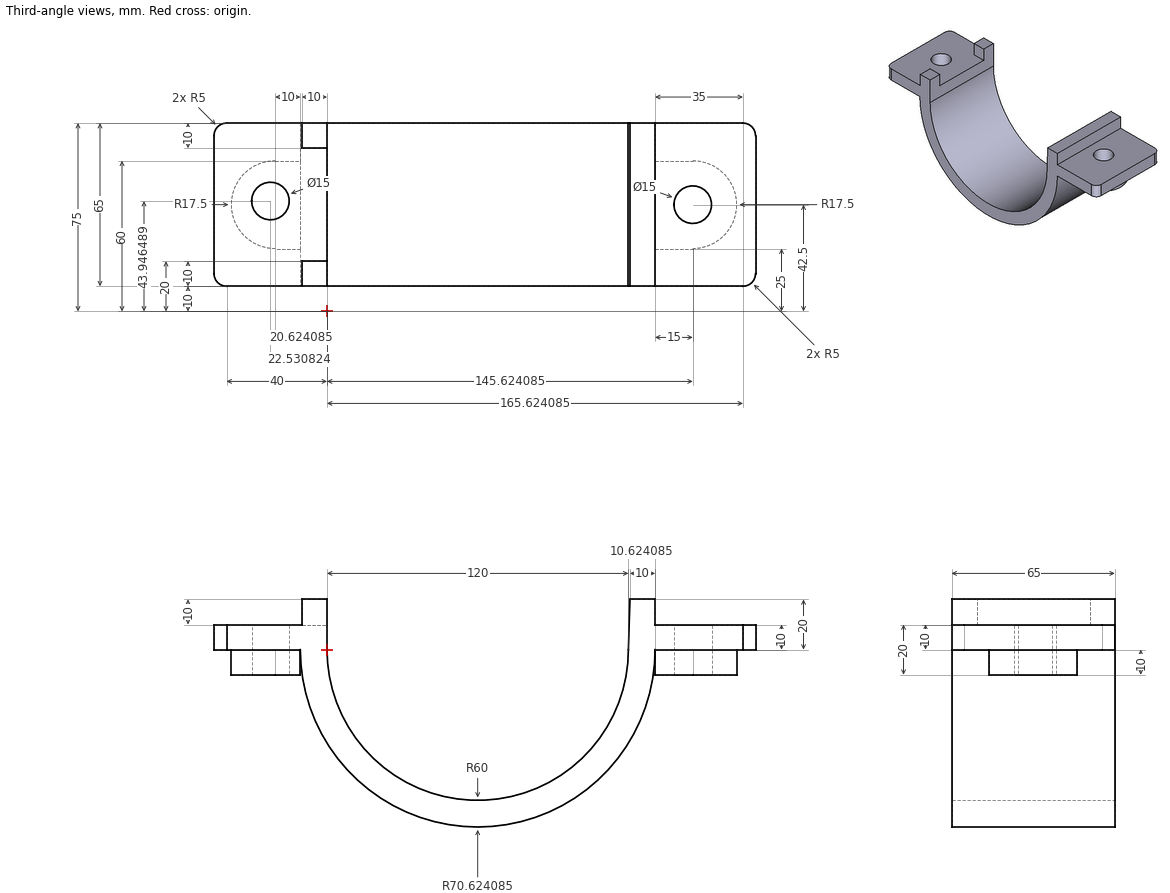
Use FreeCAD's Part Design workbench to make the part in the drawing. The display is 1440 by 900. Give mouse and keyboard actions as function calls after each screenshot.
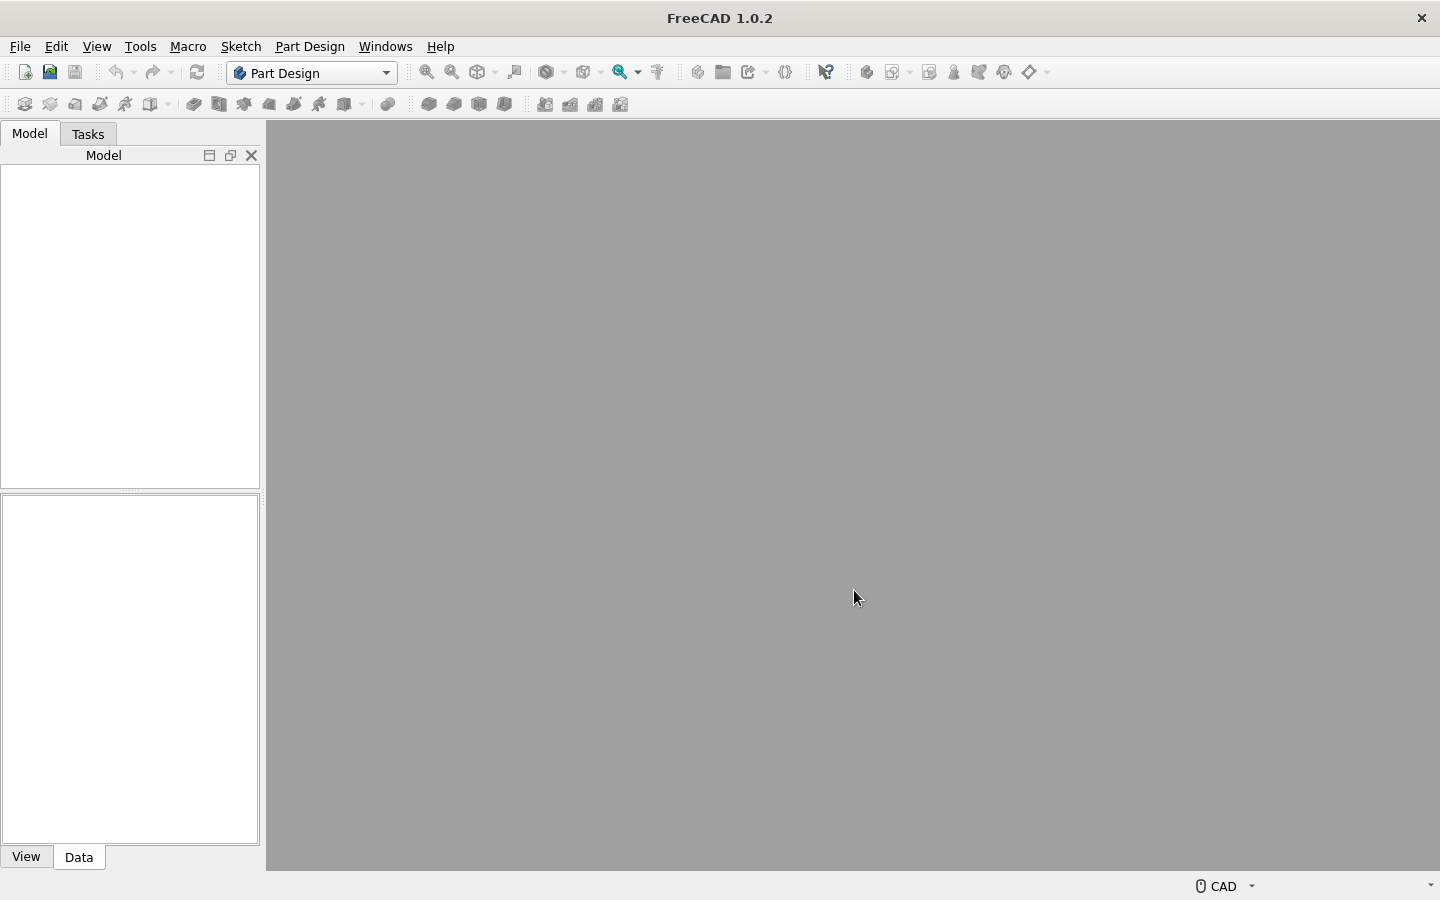
click(25, 72)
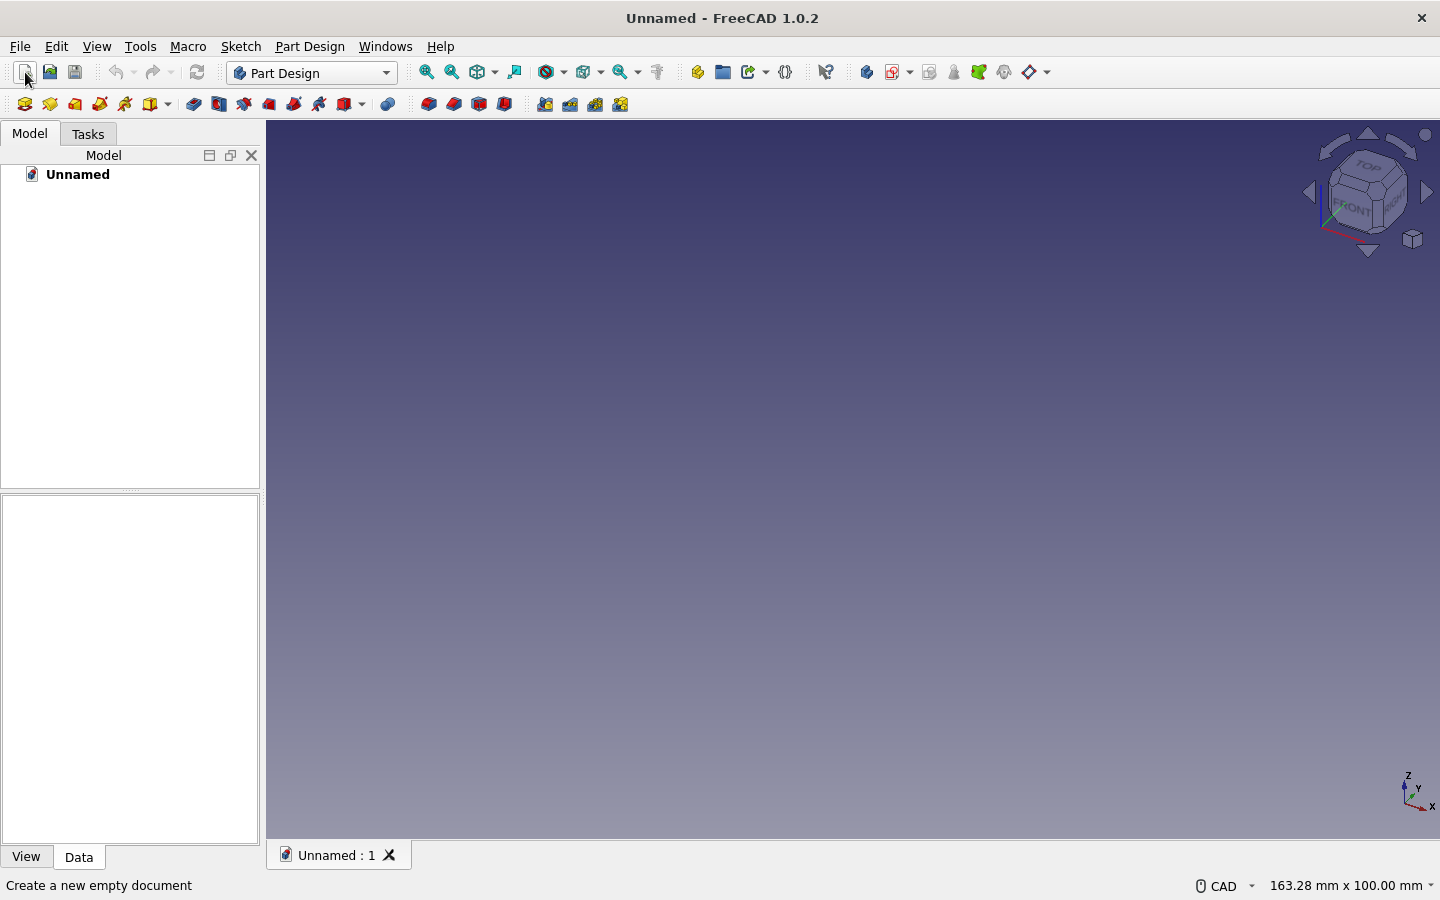
click(892, 72)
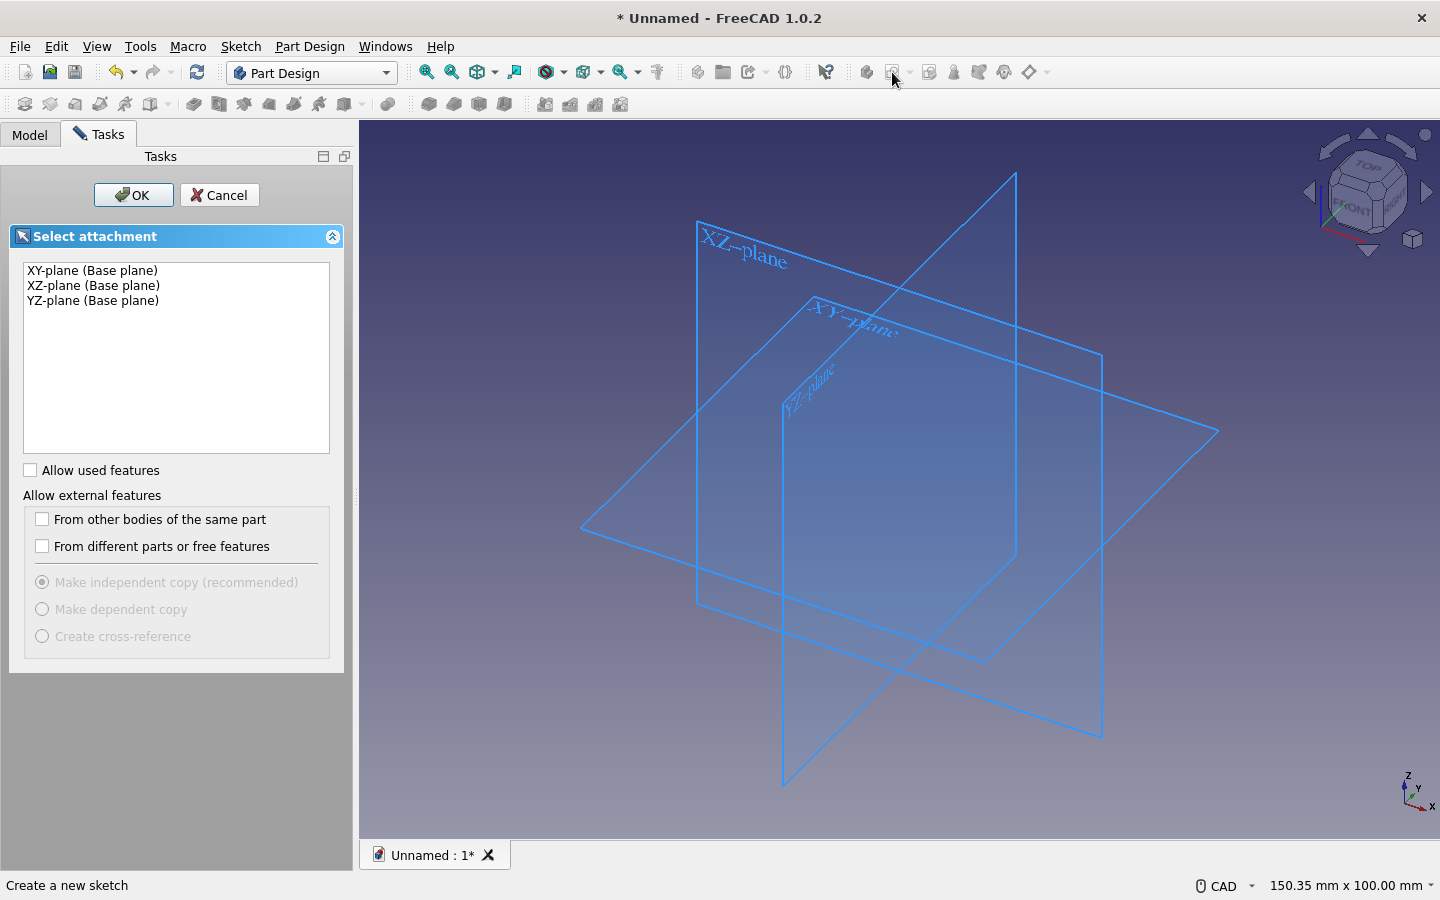
click(84, 270)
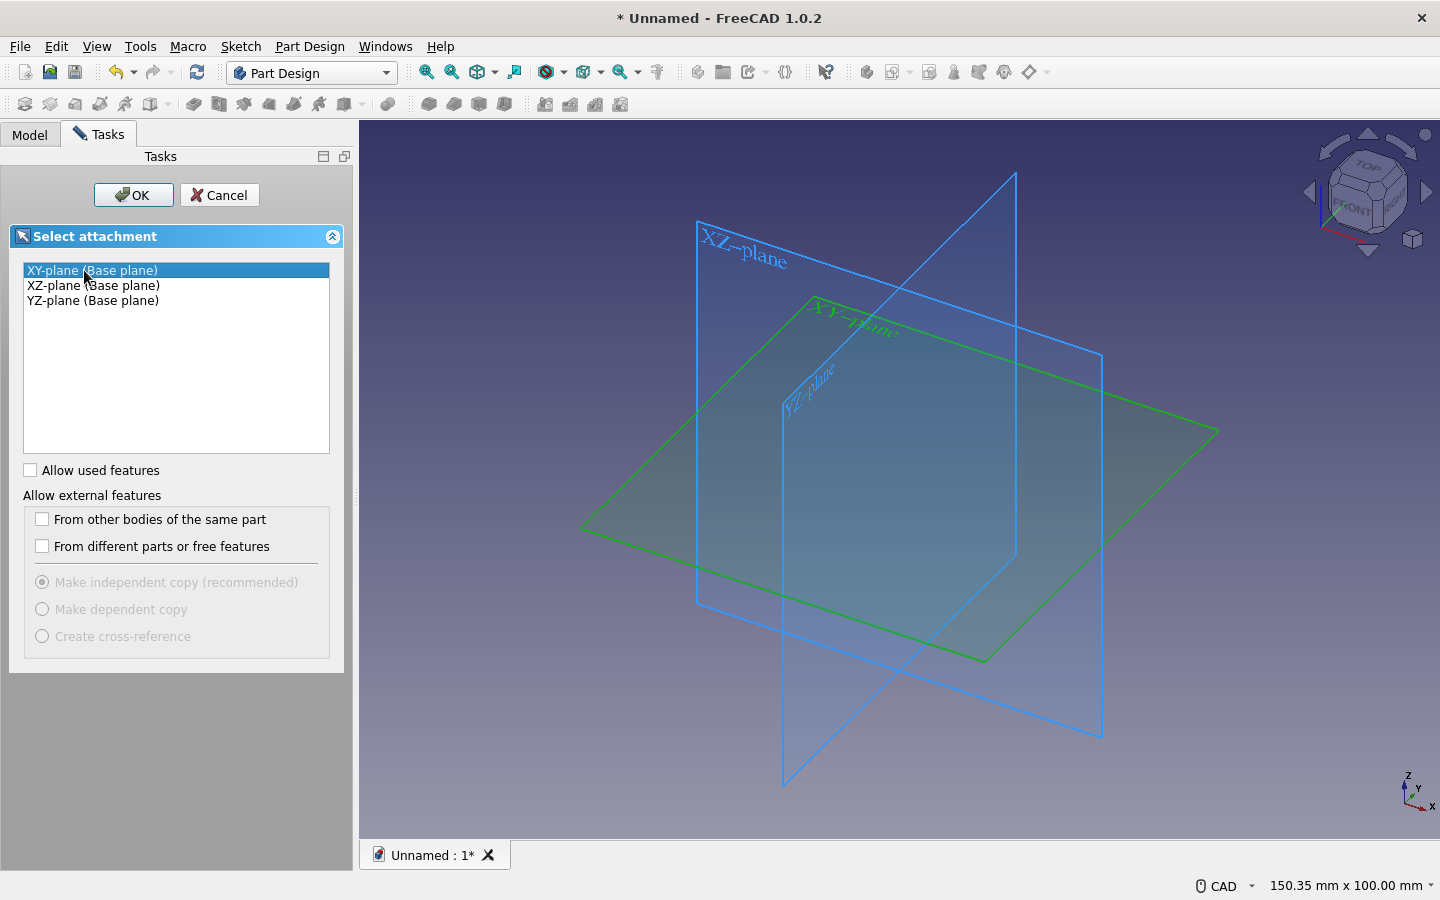
click(134, 195)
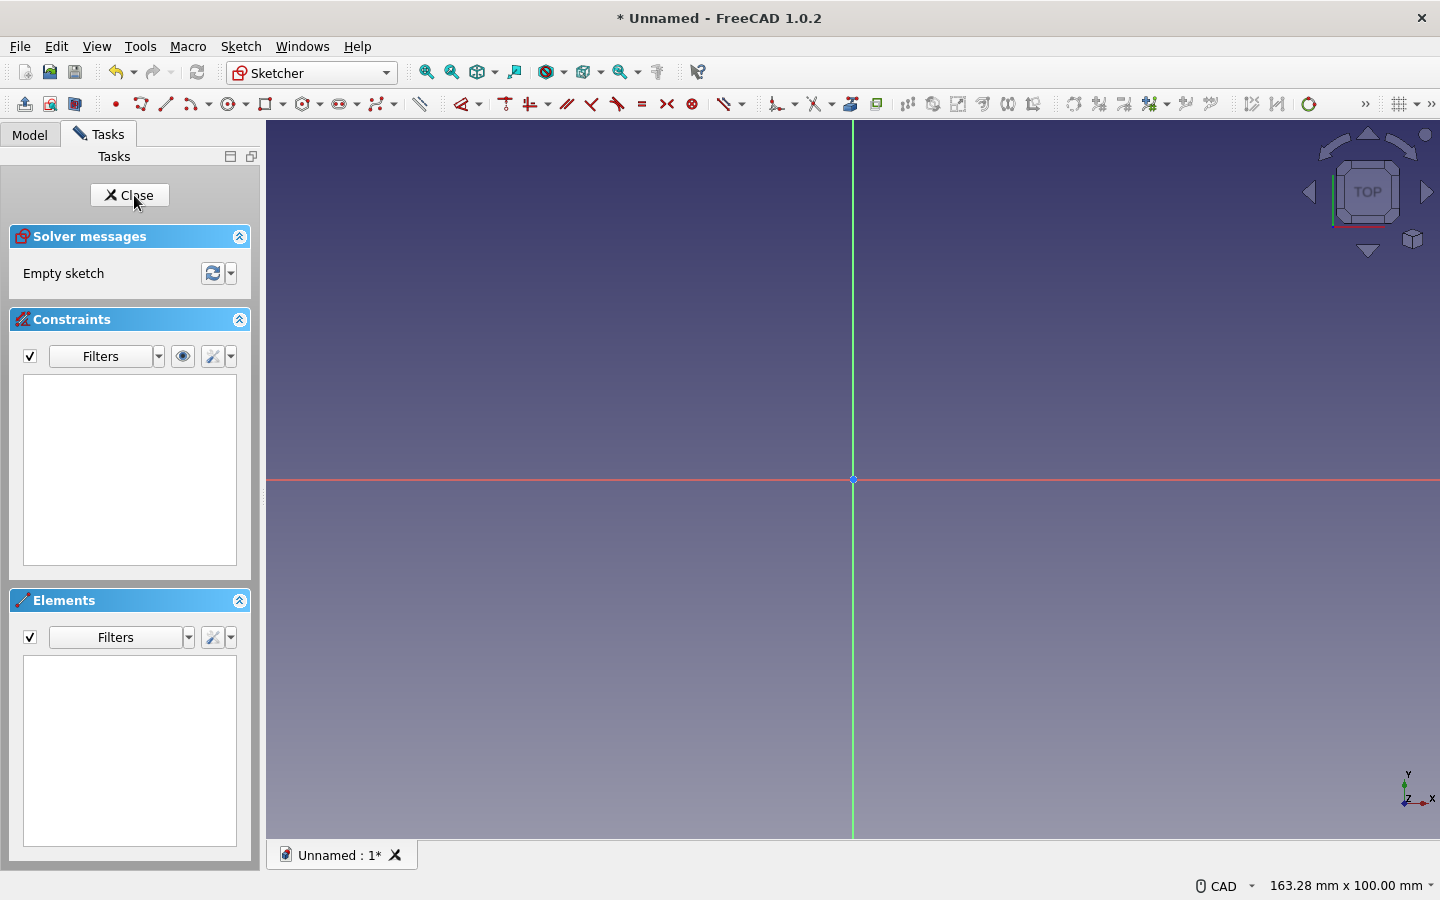
scroll(974, 811, down, 2)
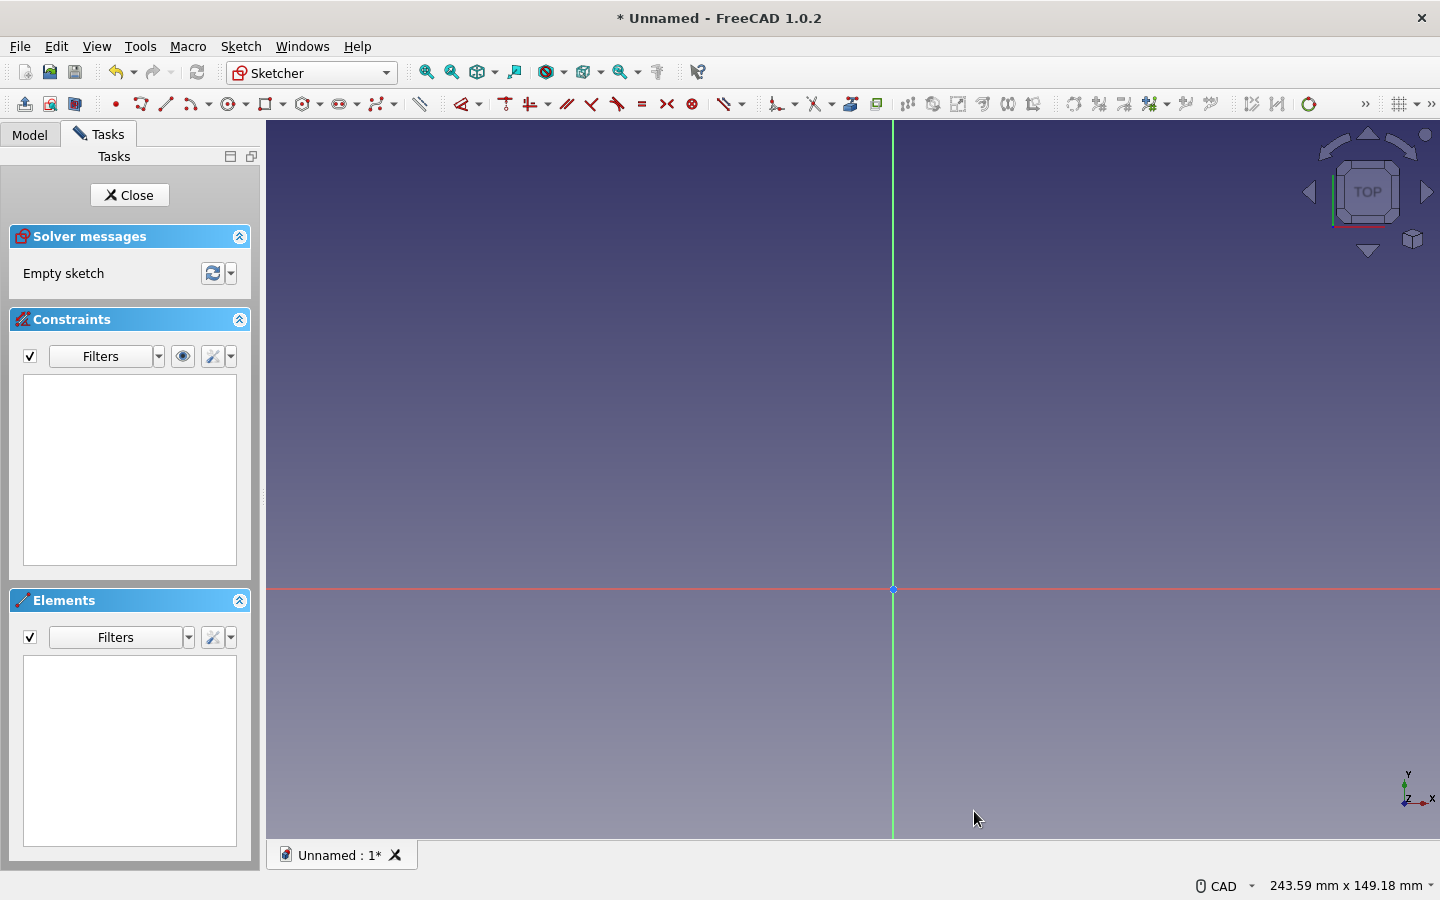
click(141, 104)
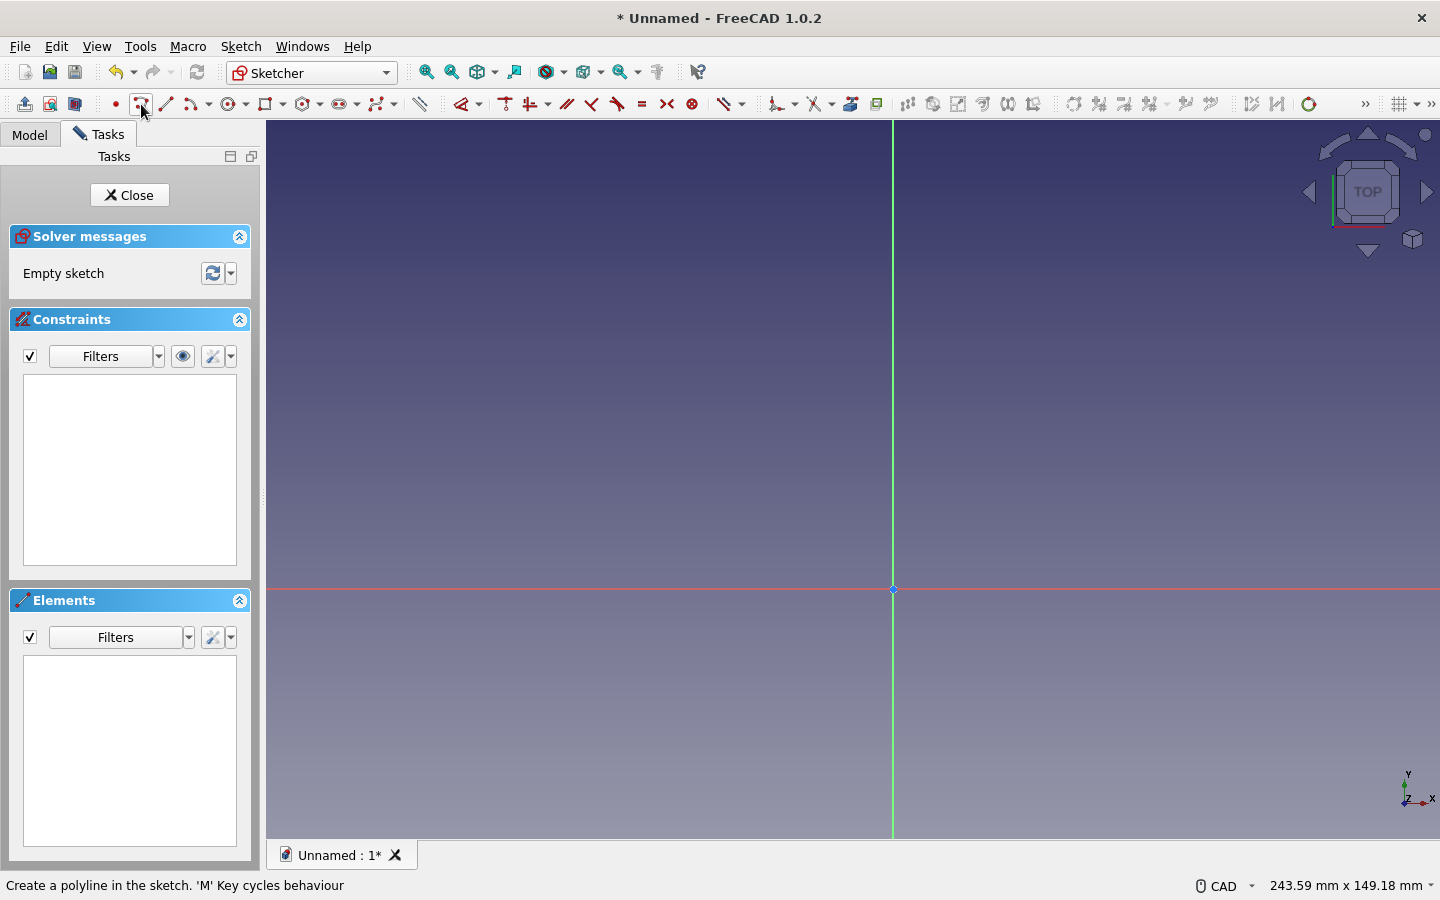
click(700, 541)
click(893, 541)
click(884, 228)
click(700, 228)
right_click(700, 228)